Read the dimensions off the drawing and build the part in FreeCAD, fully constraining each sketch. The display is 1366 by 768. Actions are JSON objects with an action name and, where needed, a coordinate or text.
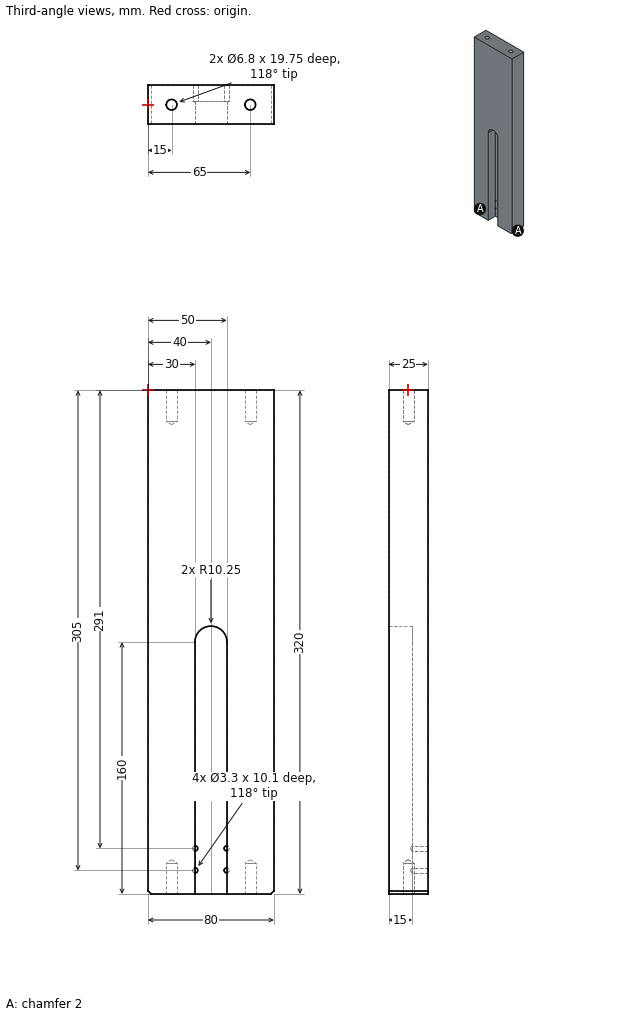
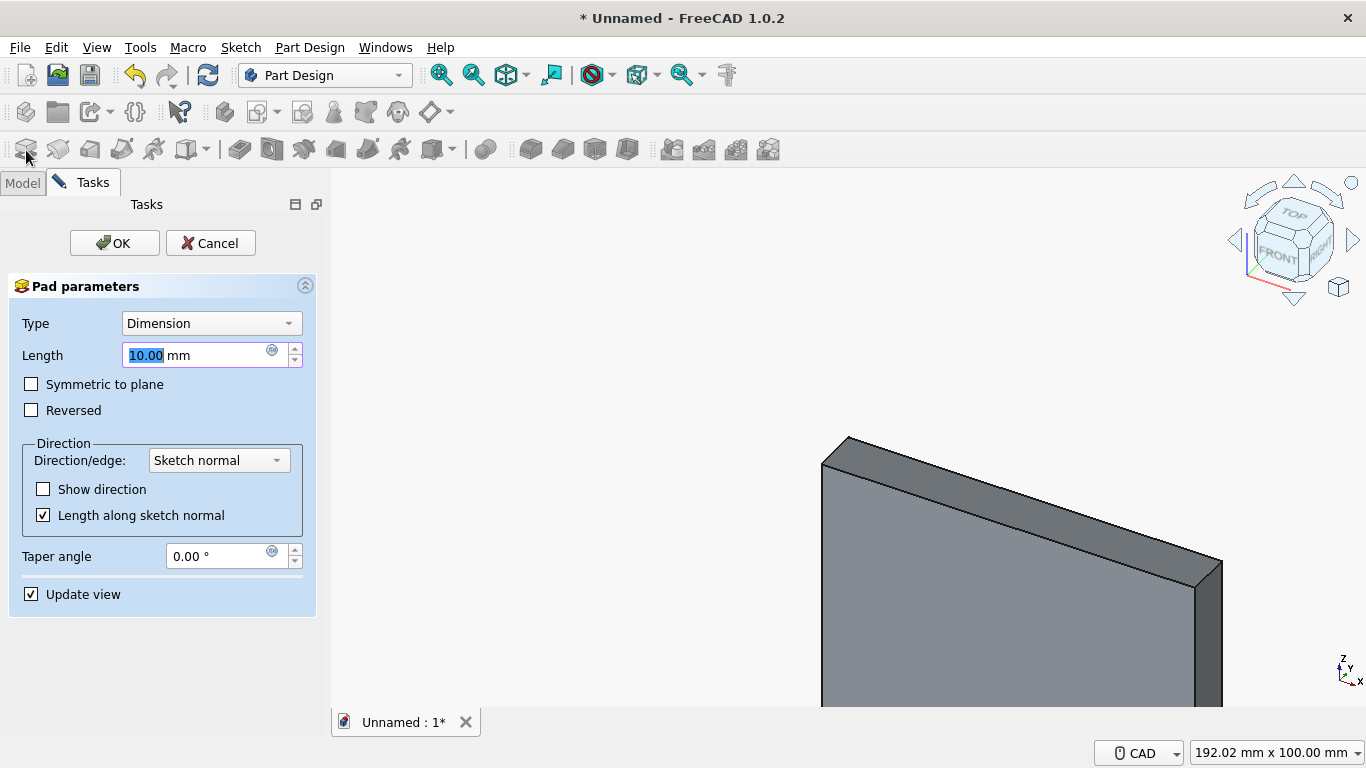
{"action": "type", "text": "25"}
{"action": "key", "text": "Tab"}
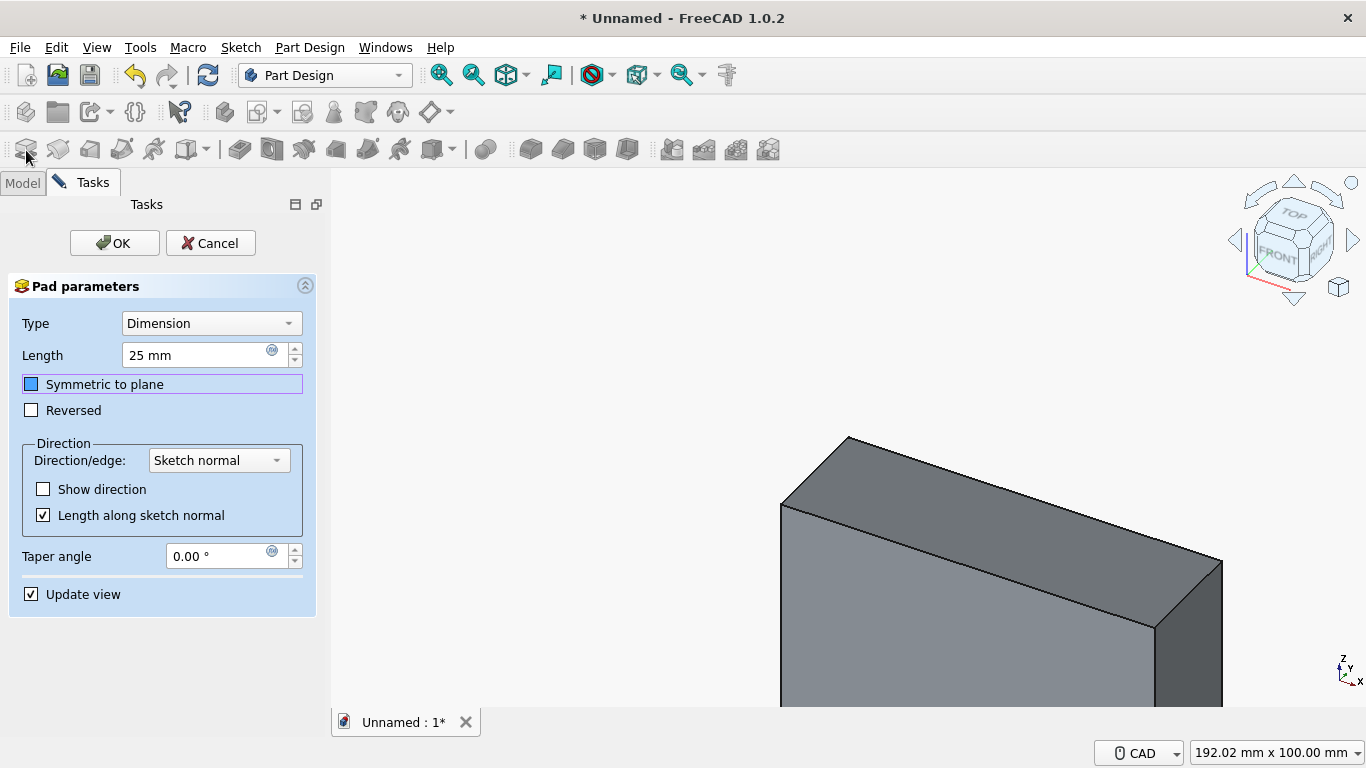
{"action": "left_click", "coordinate": [30, 384]}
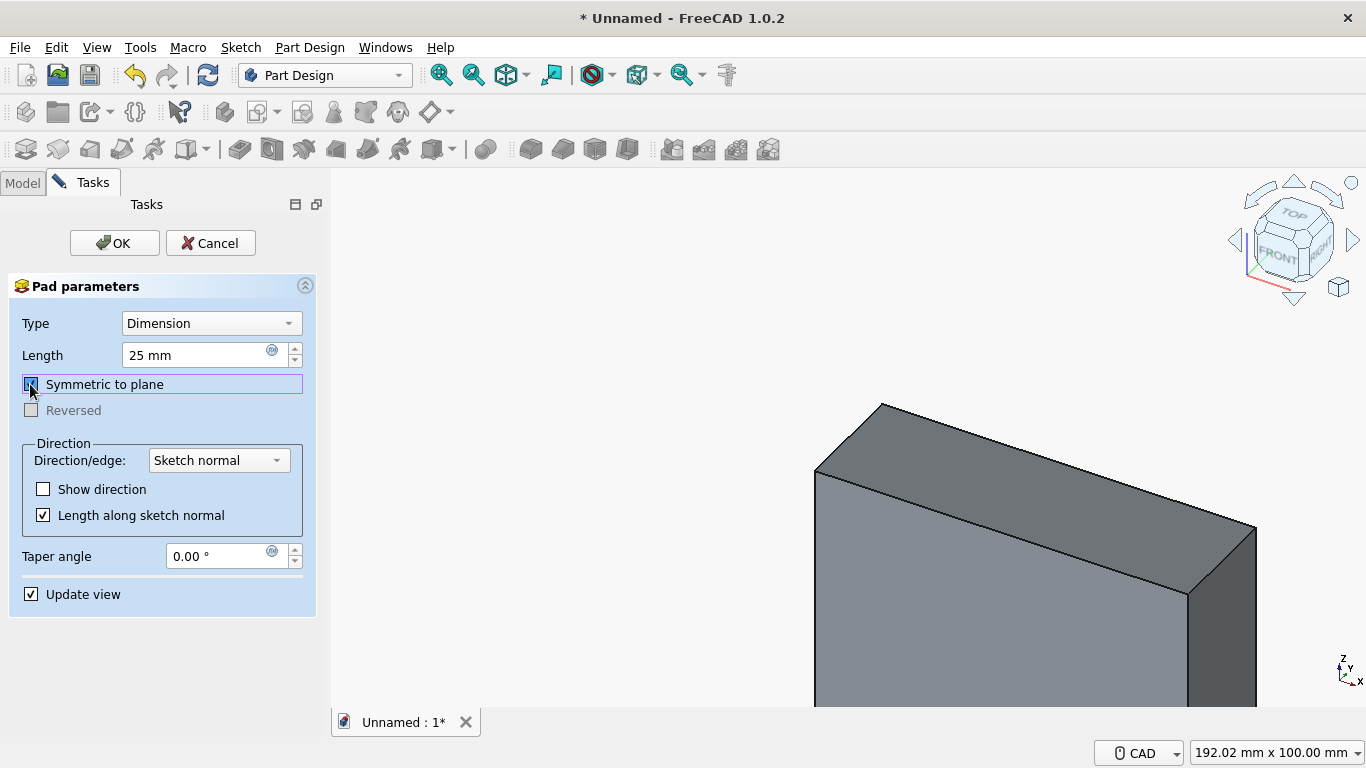
{"action": "left_click", "coordinate": [115, 243]}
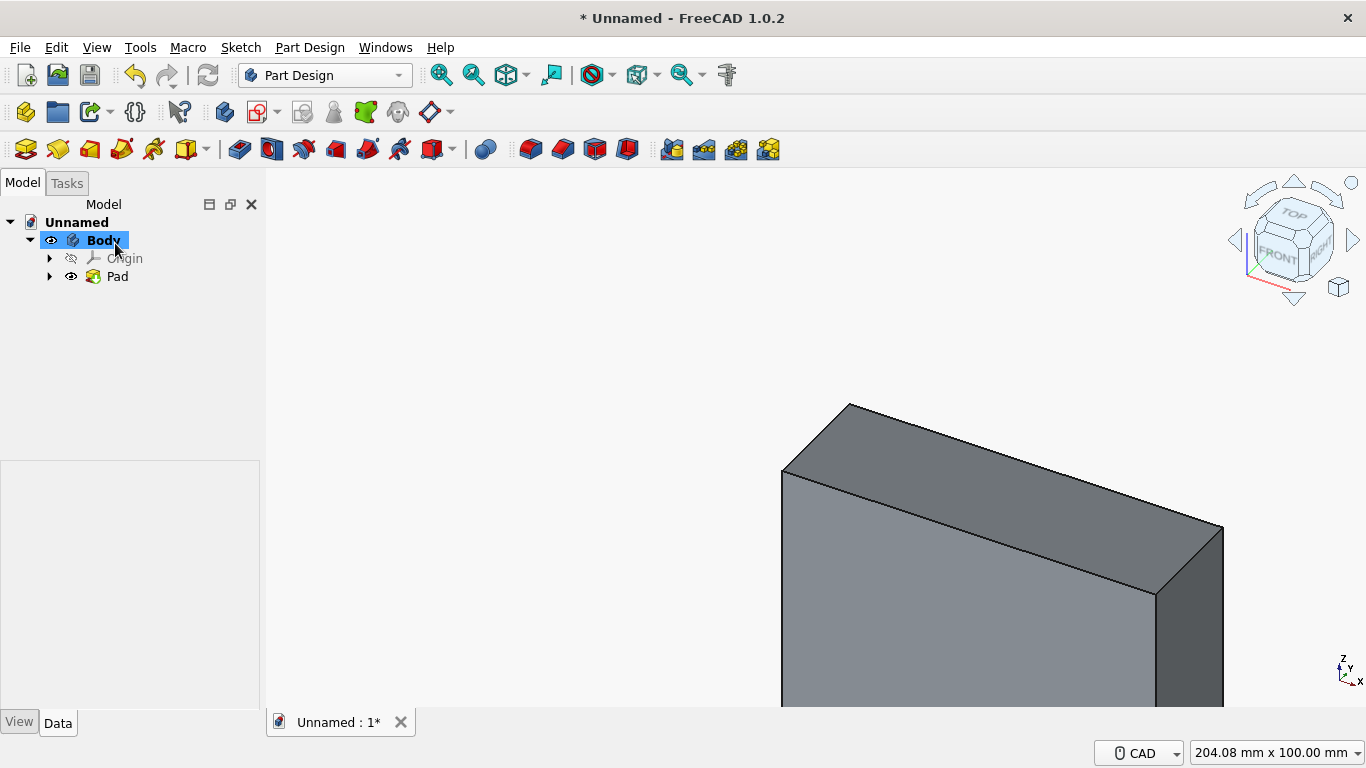
{"action": "left_click", "coordinate": [442, 76]}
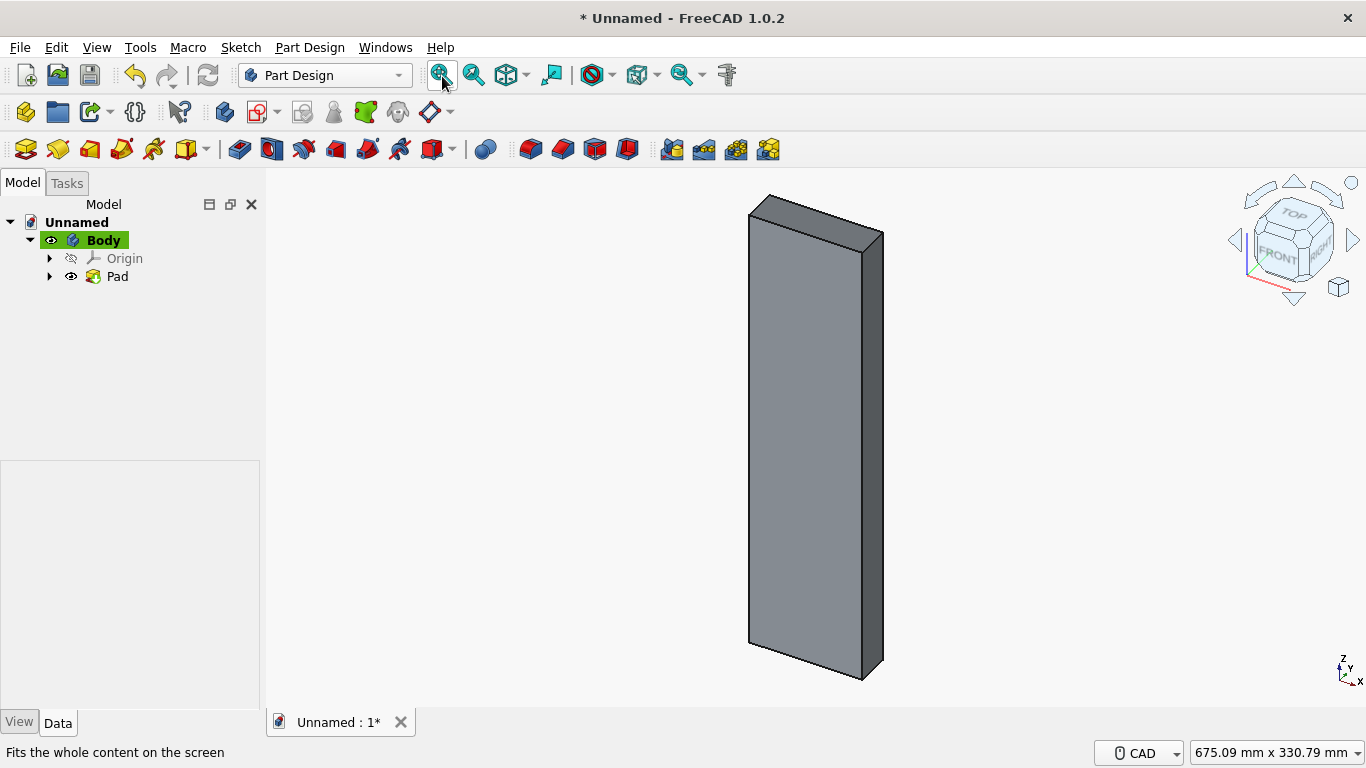
{"action": "left_click", "coordinate": [848, 234]}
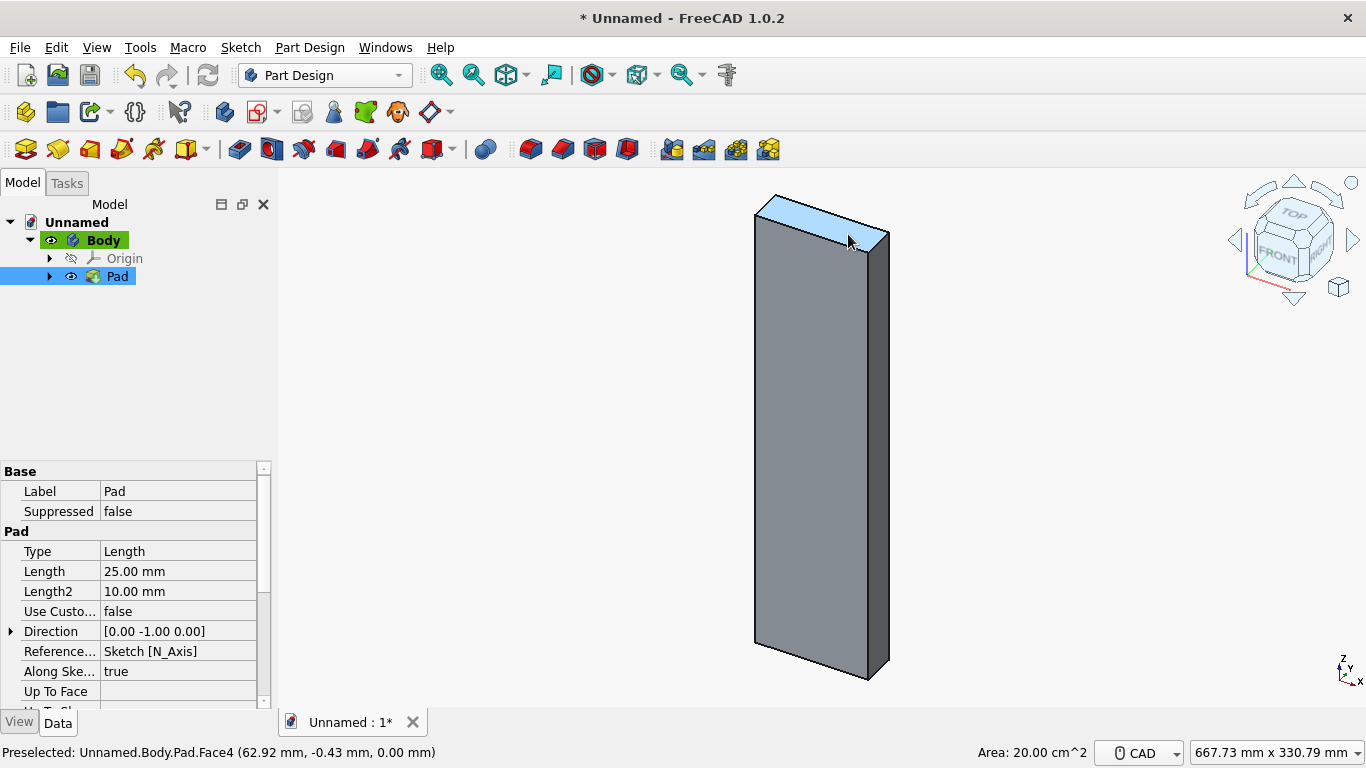
{"action": "left_click", "coordinate": [258, 112]}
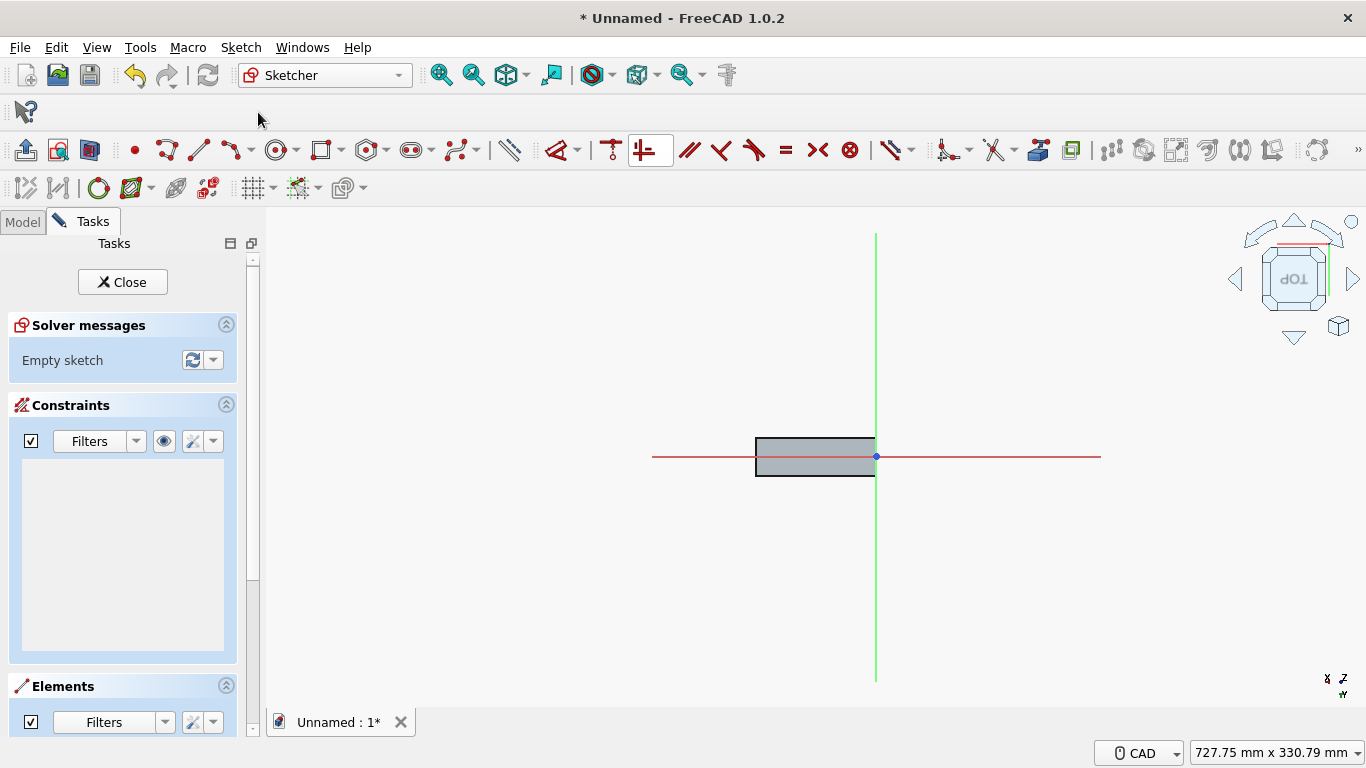
{"action": "scroll", "coordinate": [840, 457], "scroll_direction": "up", "scroll_amount": 9}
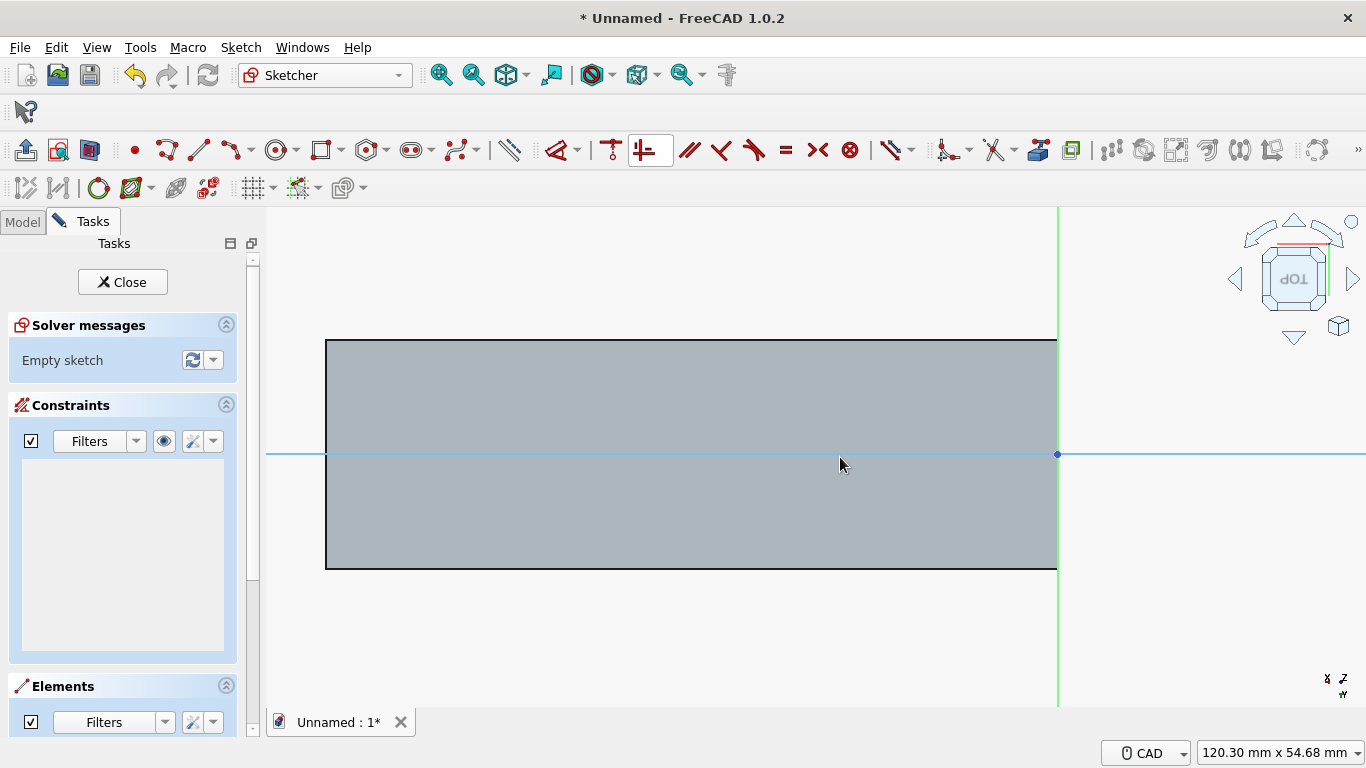
{"action": "key", "text": "g c"}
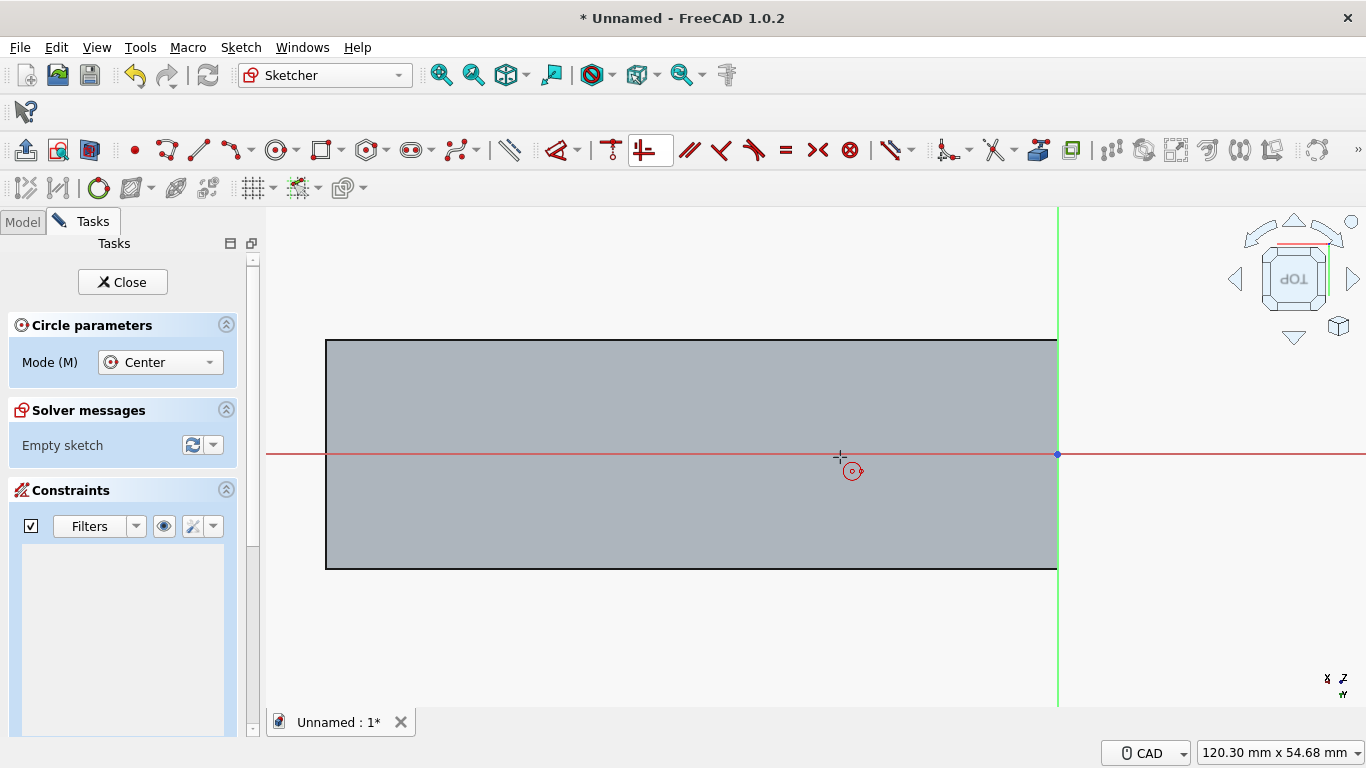
{"action": "left_click", "coordinate": [921, 454]}
{"action": "mouse_move", "coordinate": [943, 432]}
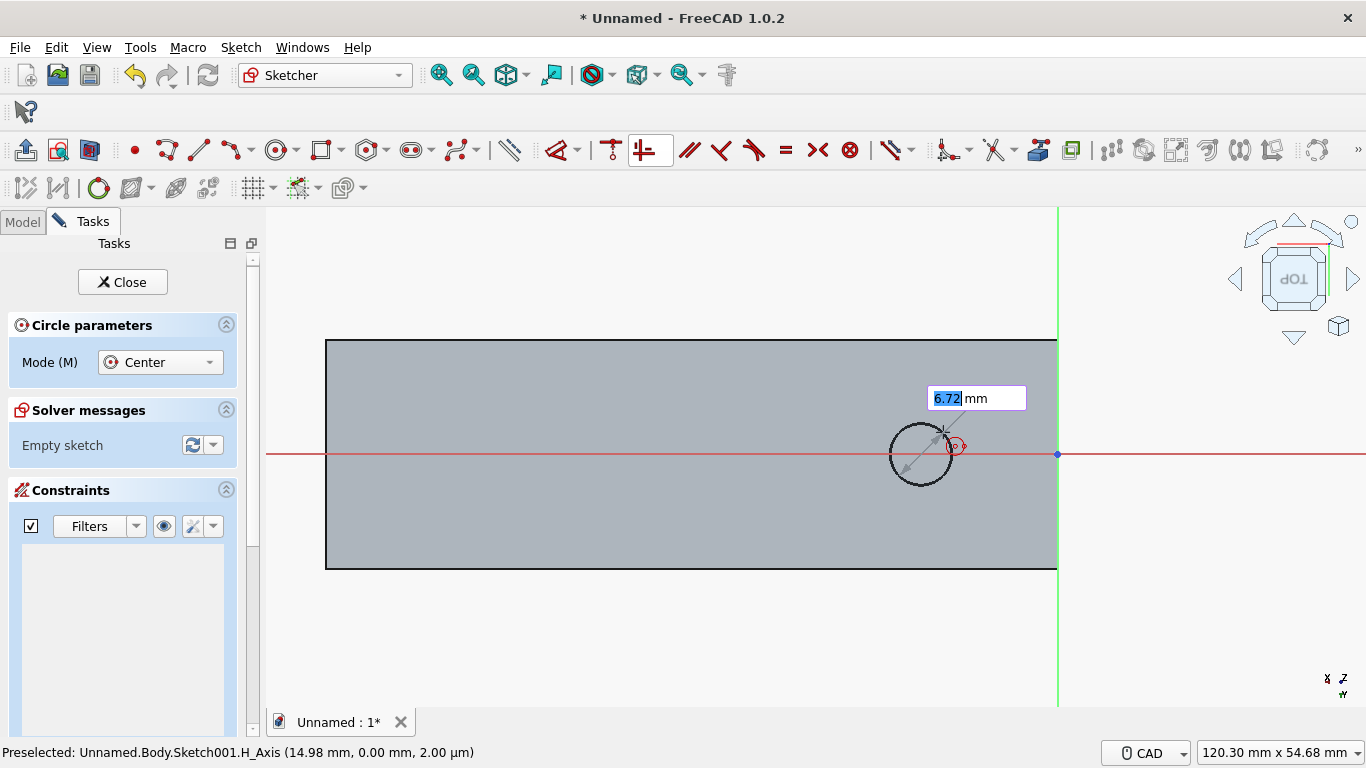
{"action": "type", "text": "6.8"}
{"action": "key", "text": "Return"}